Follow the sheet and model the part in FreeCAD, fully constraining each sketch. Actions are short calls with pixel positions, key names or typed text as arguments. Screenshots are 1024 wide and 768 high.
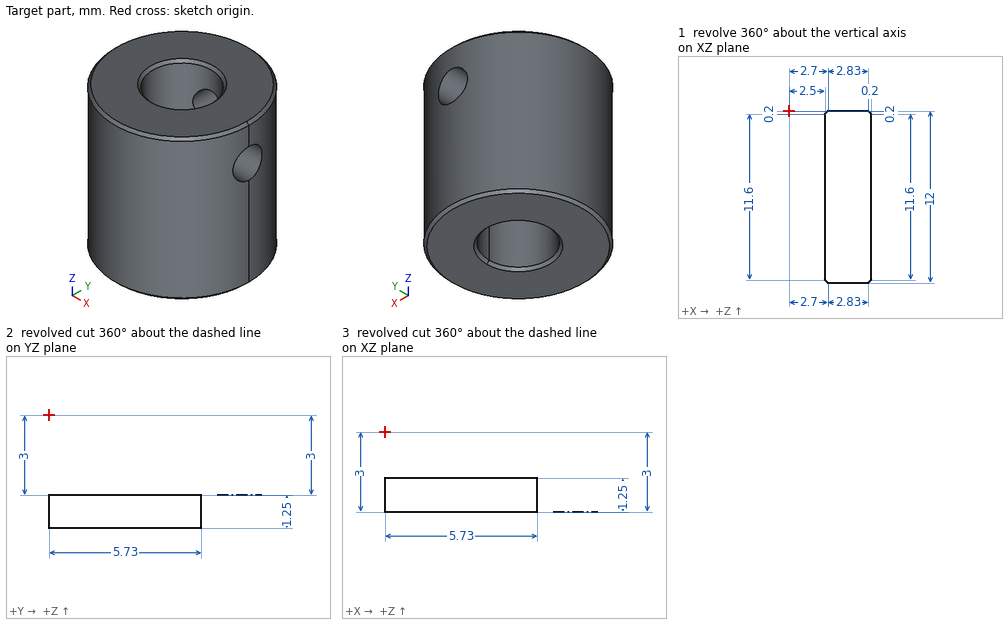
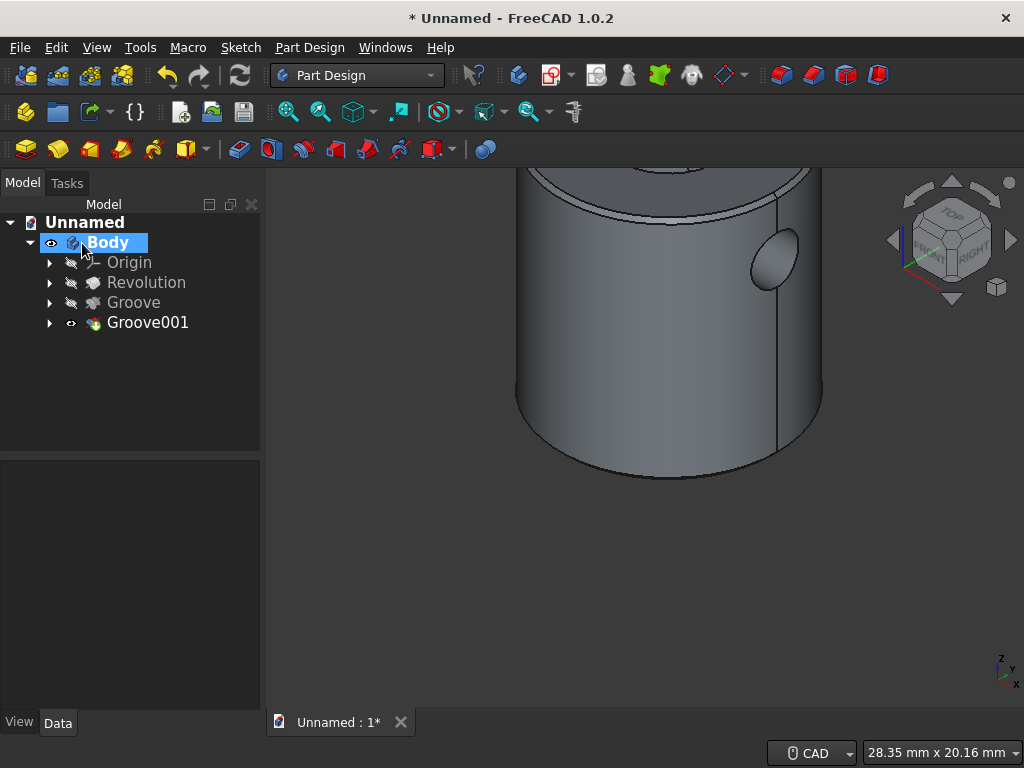
click(290, 112)